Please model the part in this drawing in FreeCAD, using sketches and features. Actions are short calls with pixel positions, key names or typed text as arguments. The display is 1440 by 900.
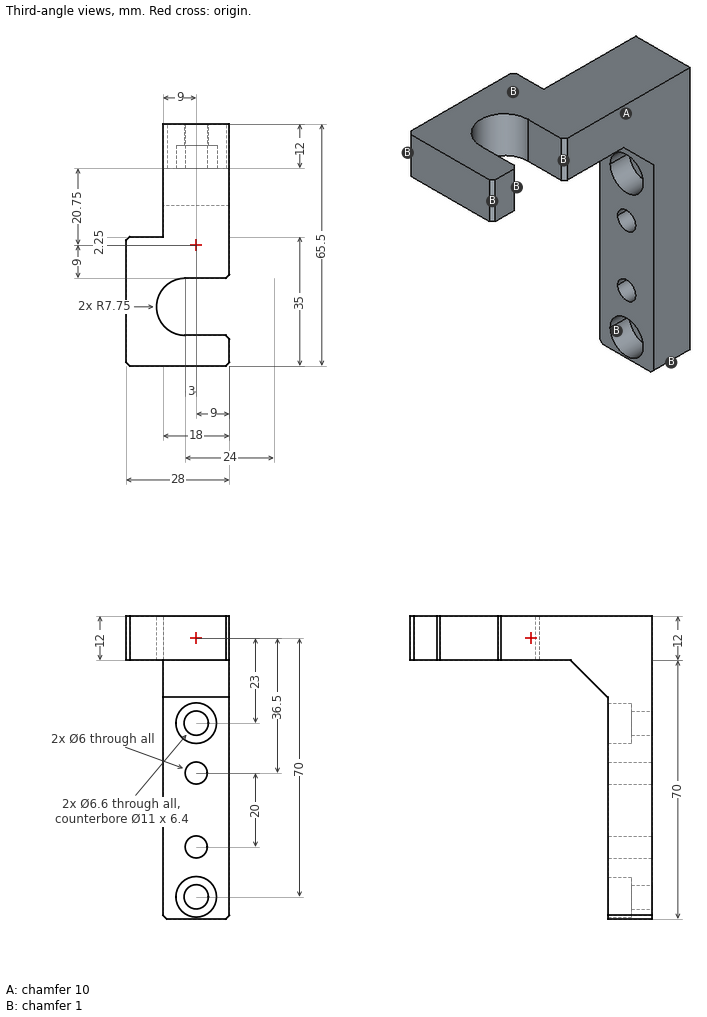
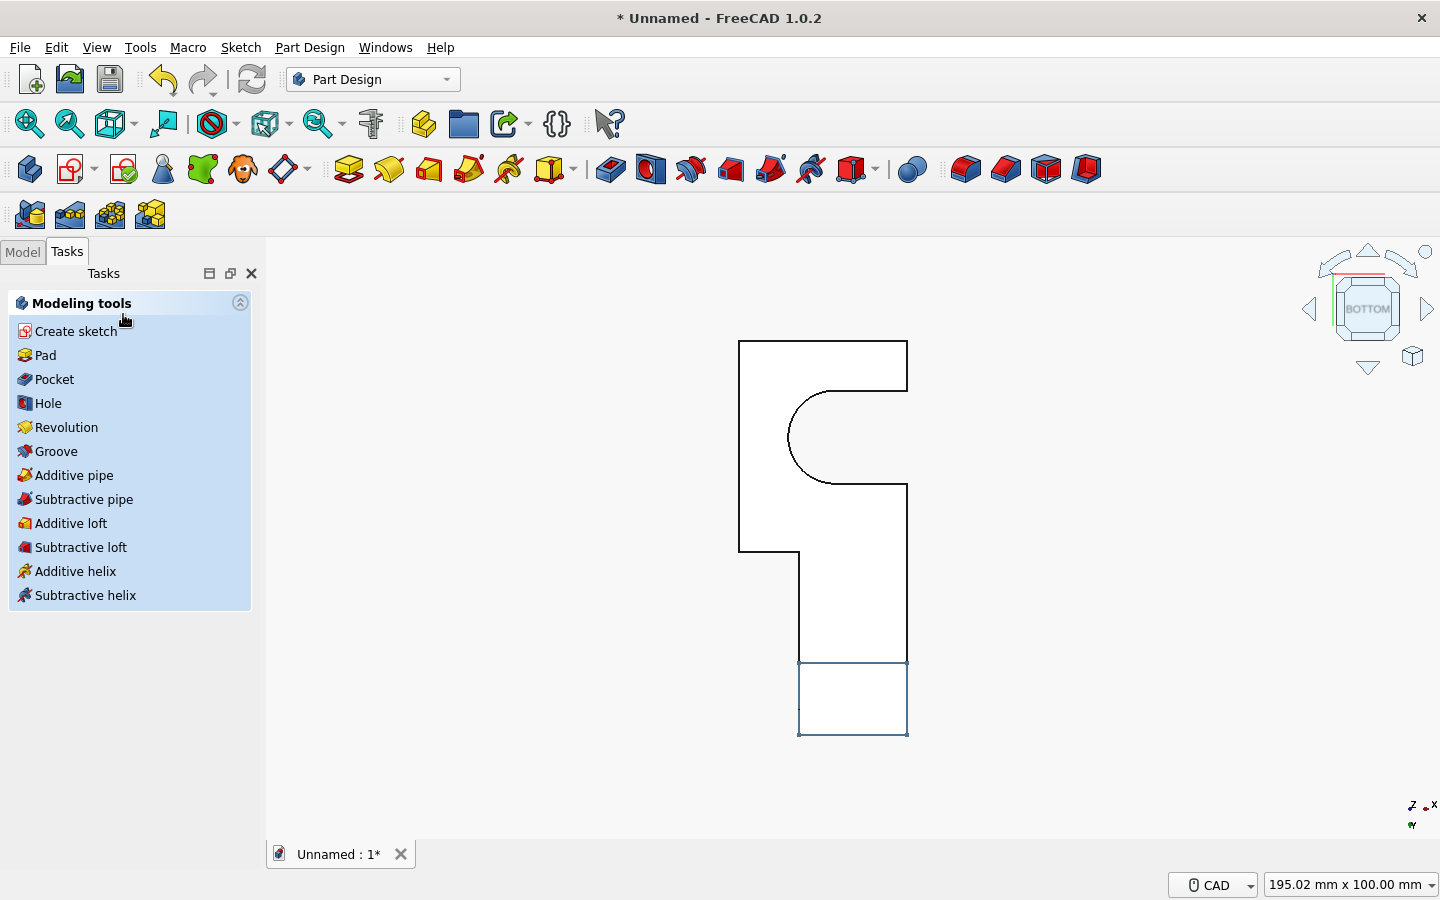
click(350, 170)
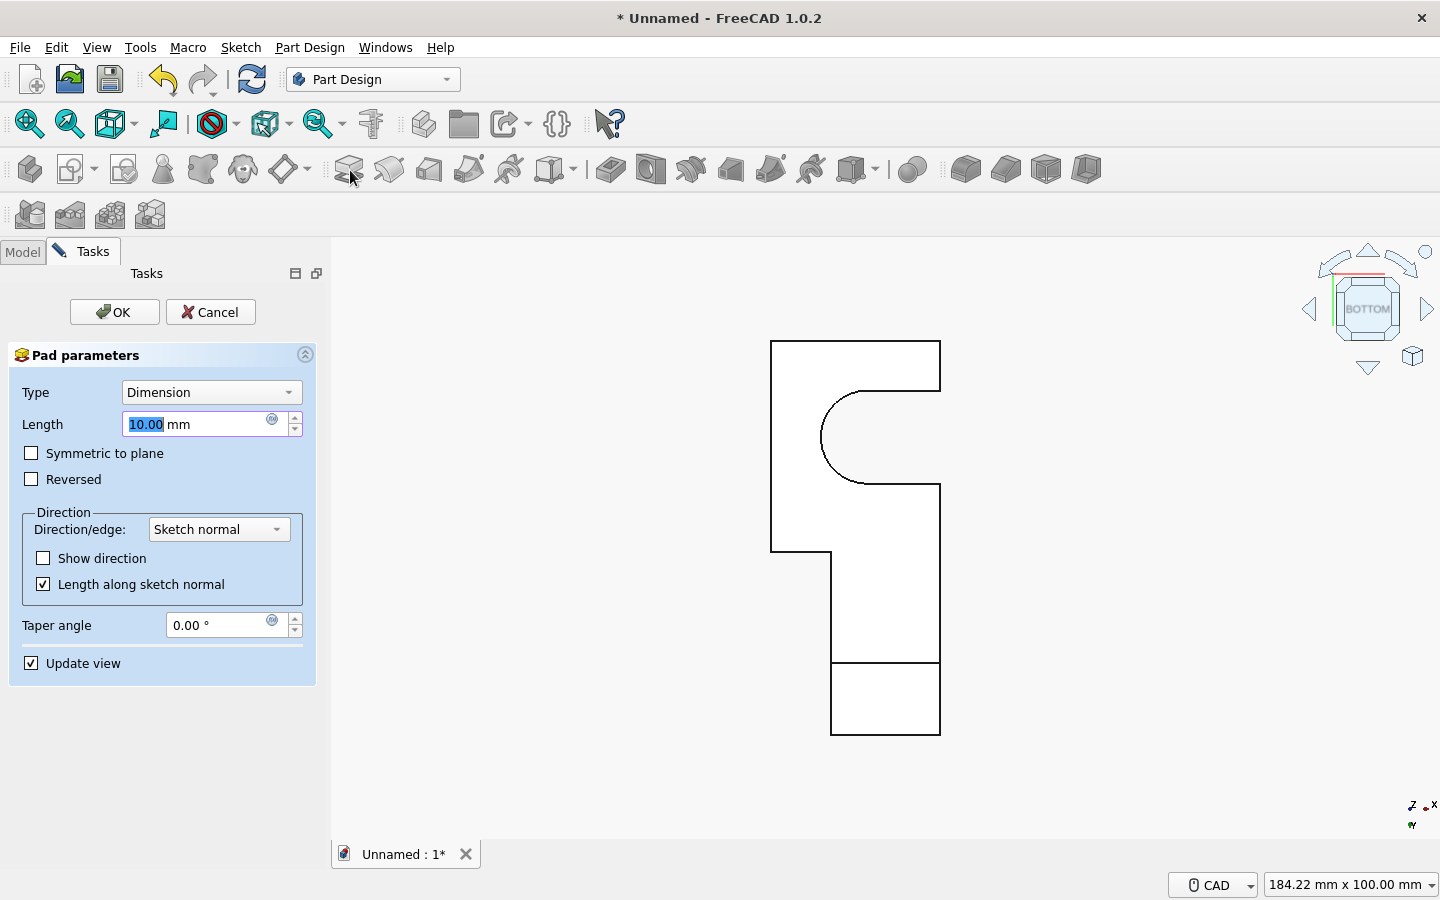
text(70)
key(Tab)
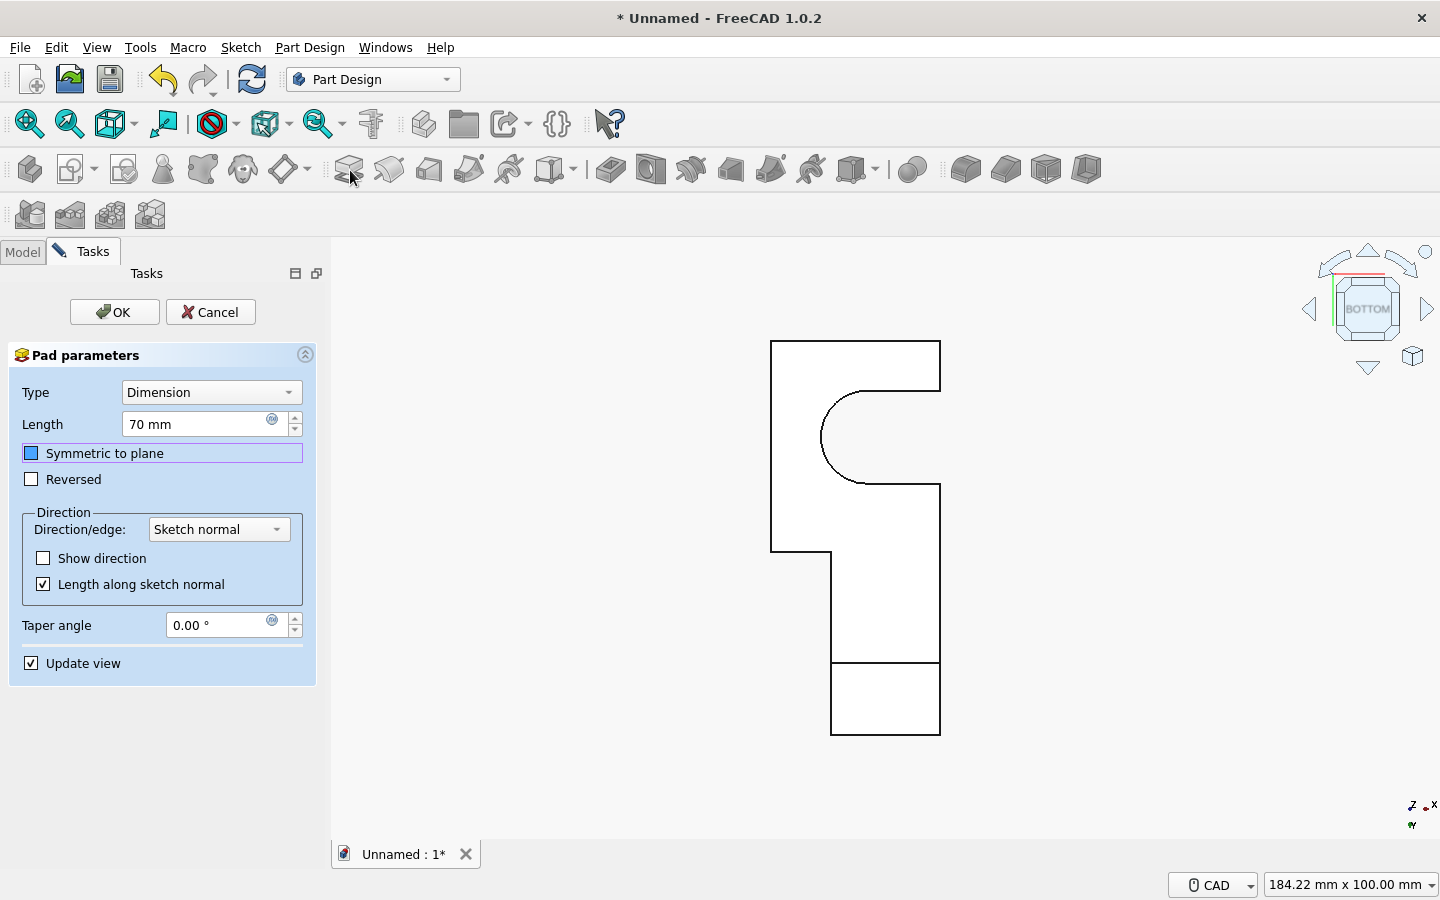
click(115, 312)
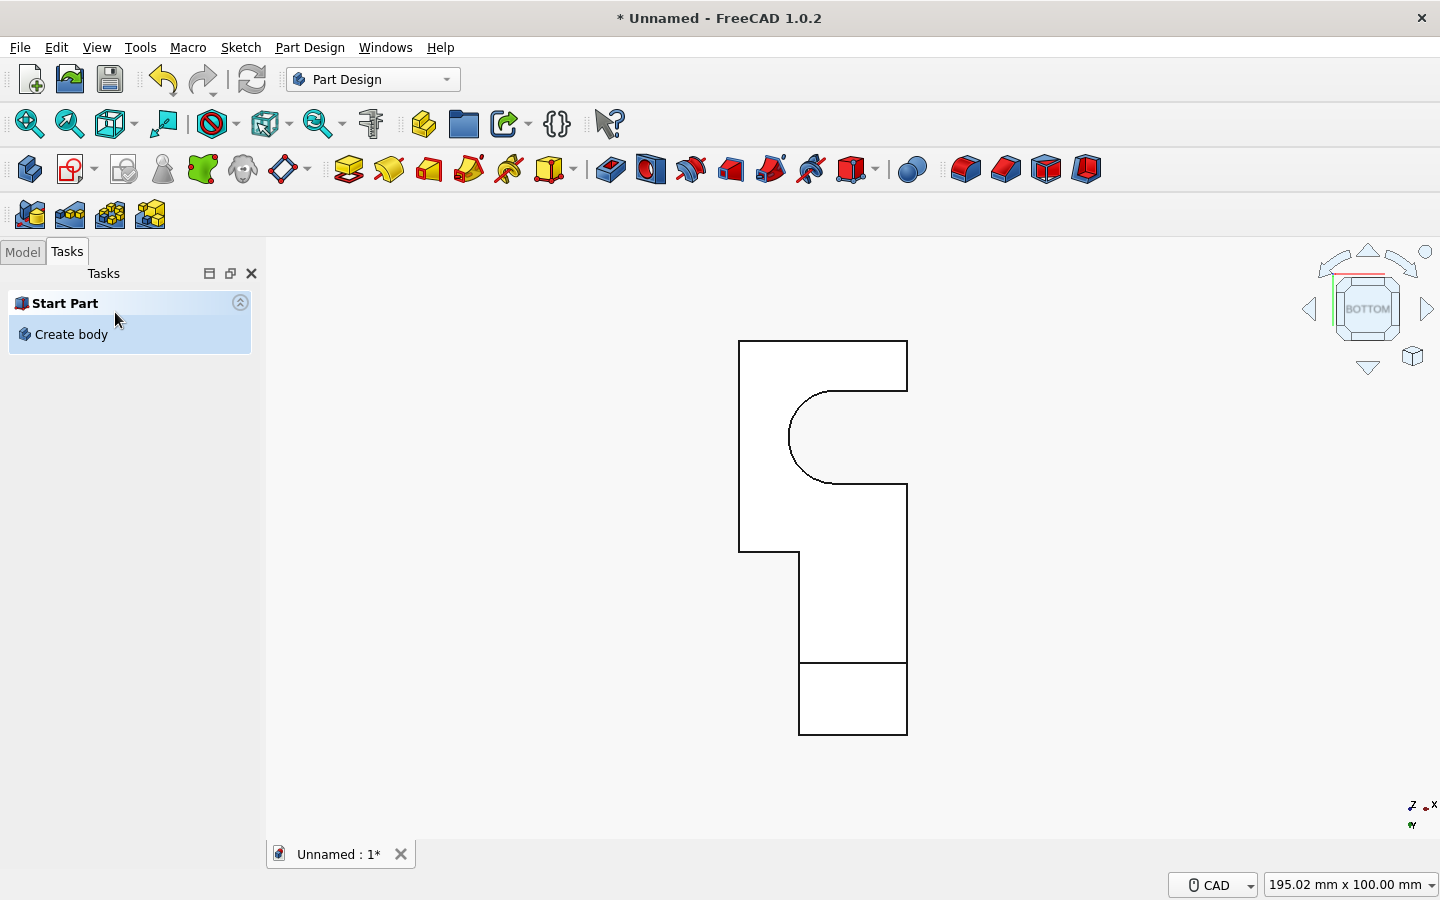
key(0)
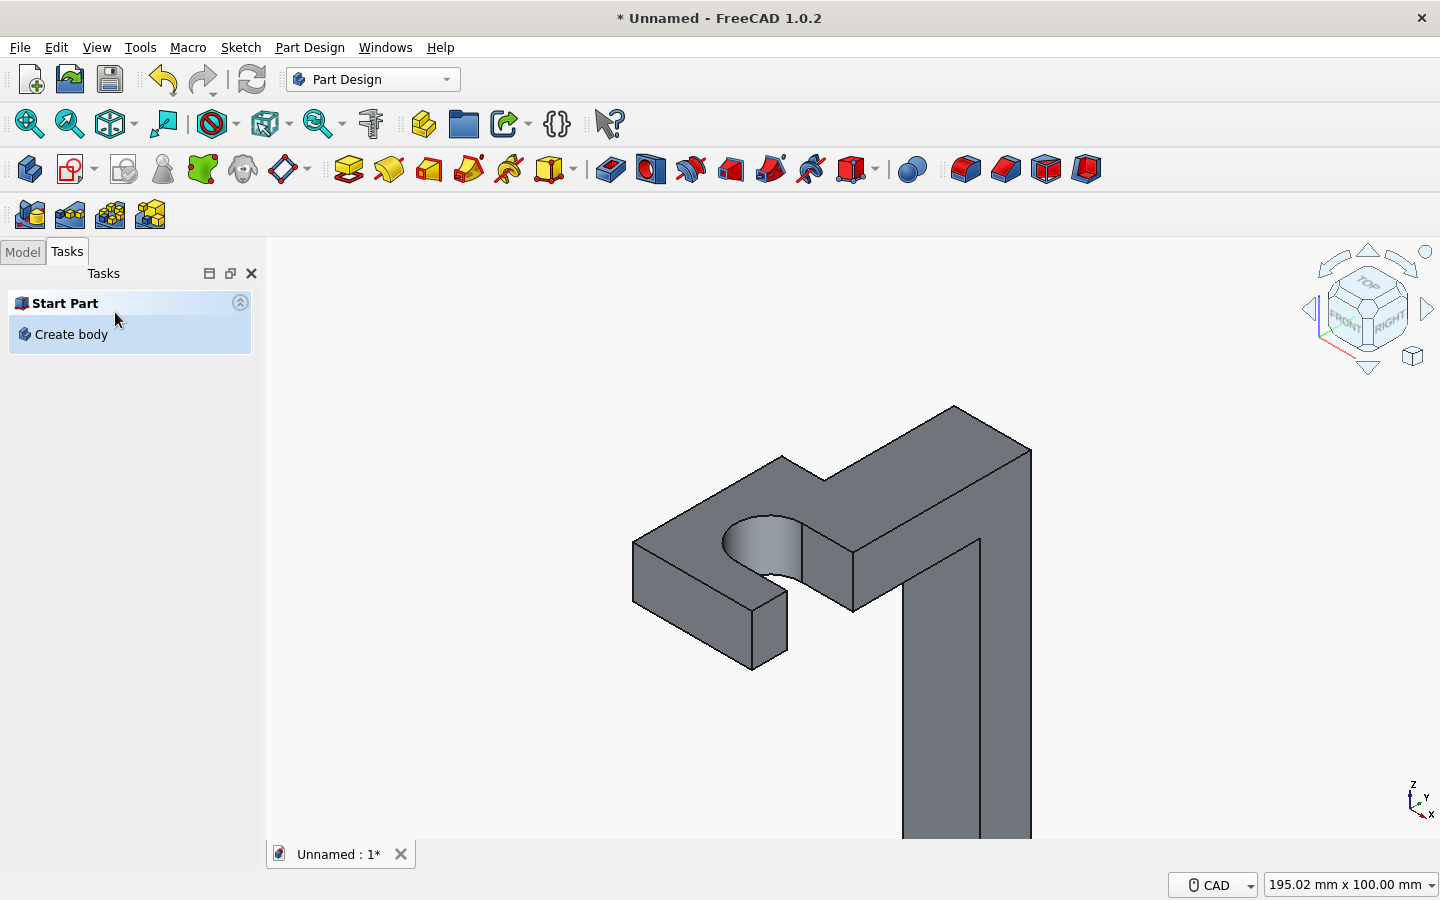
click(30, 124)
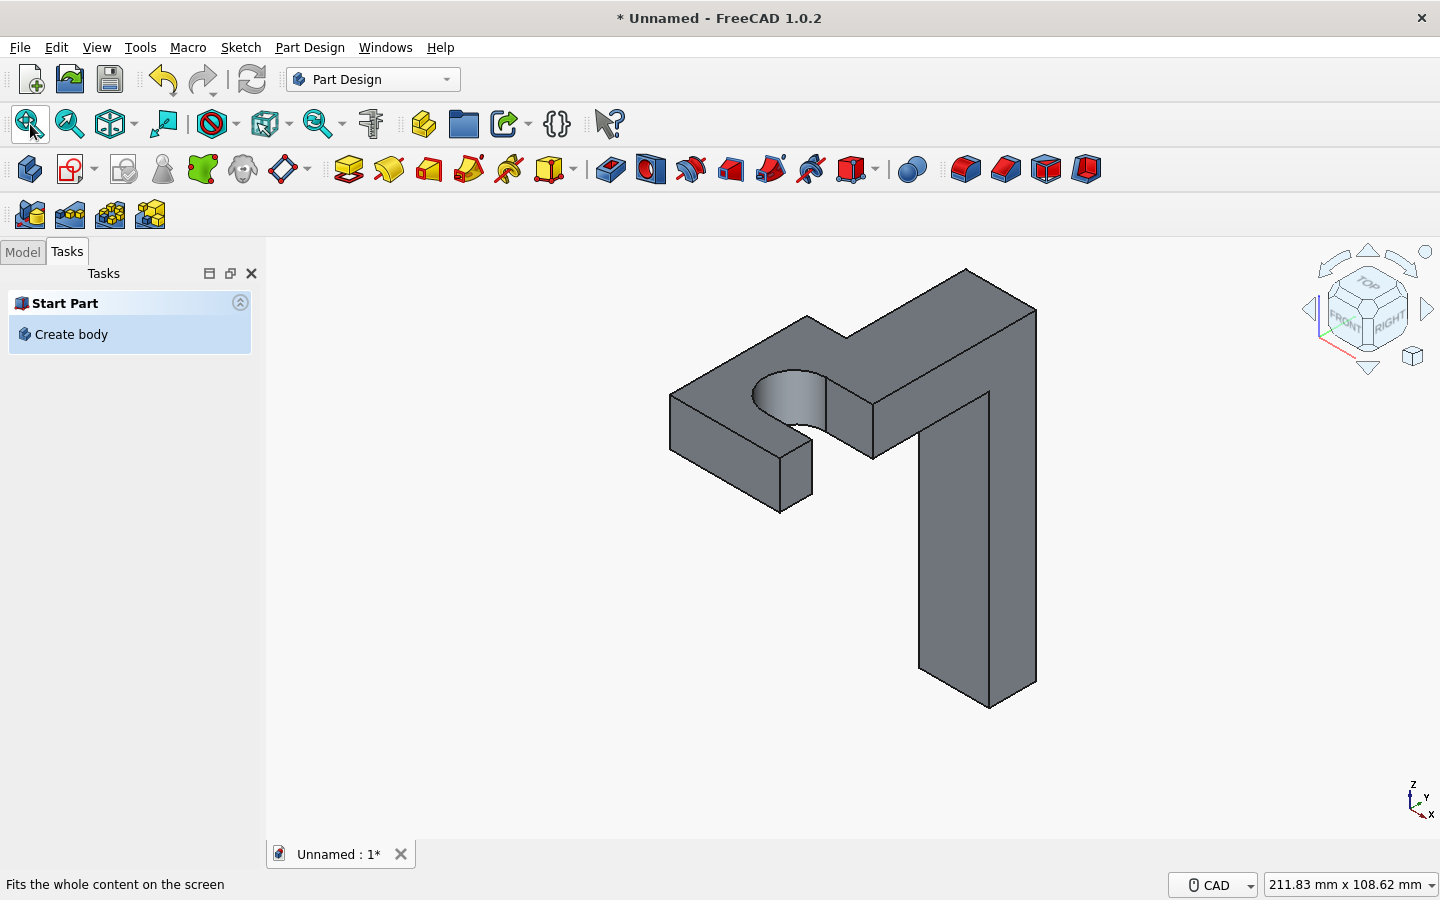
key(2)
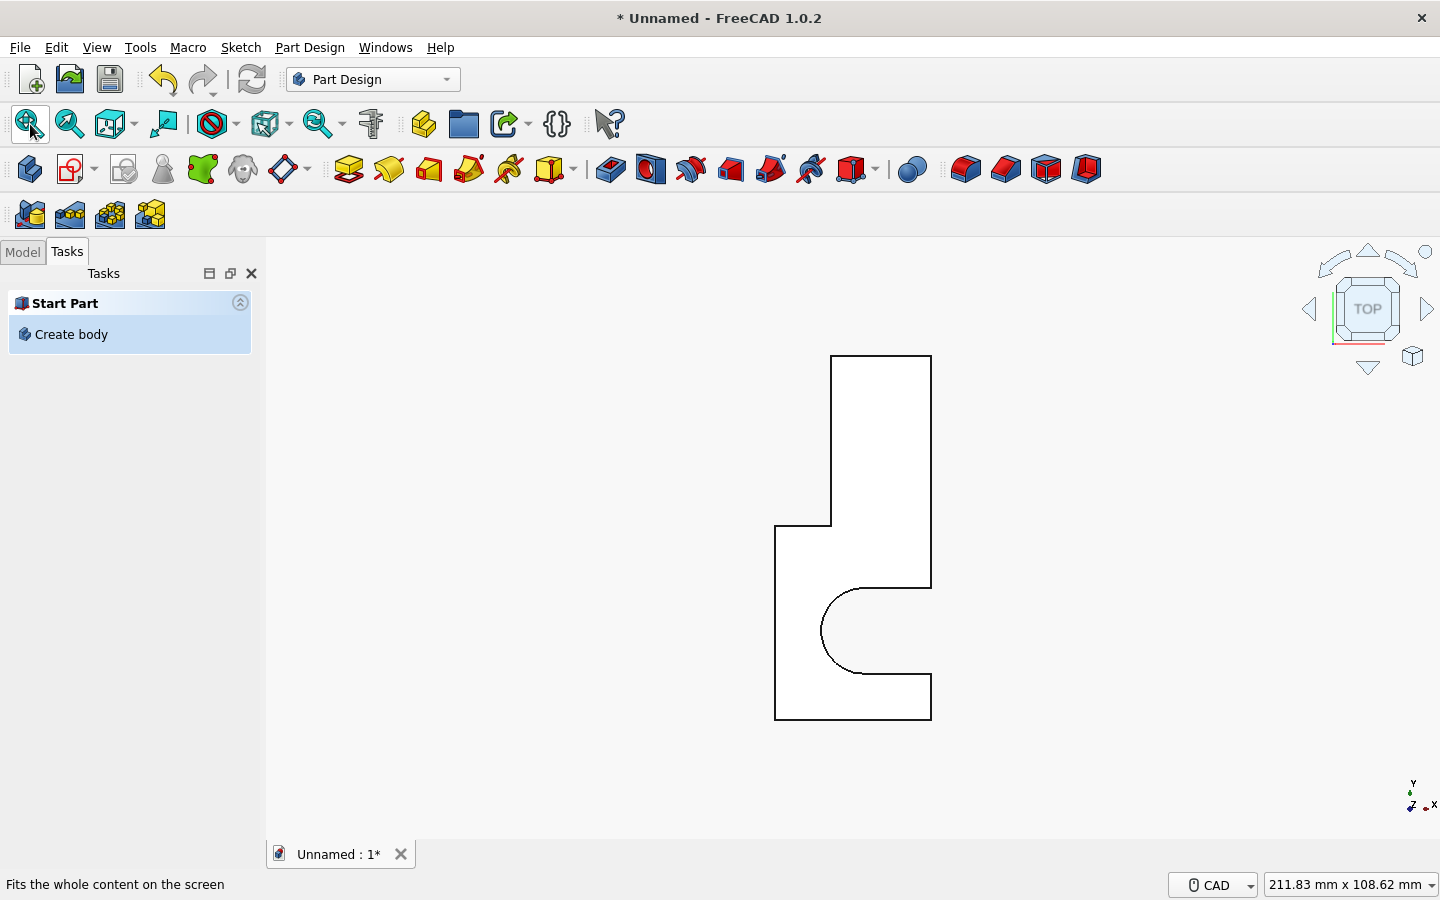
key(1)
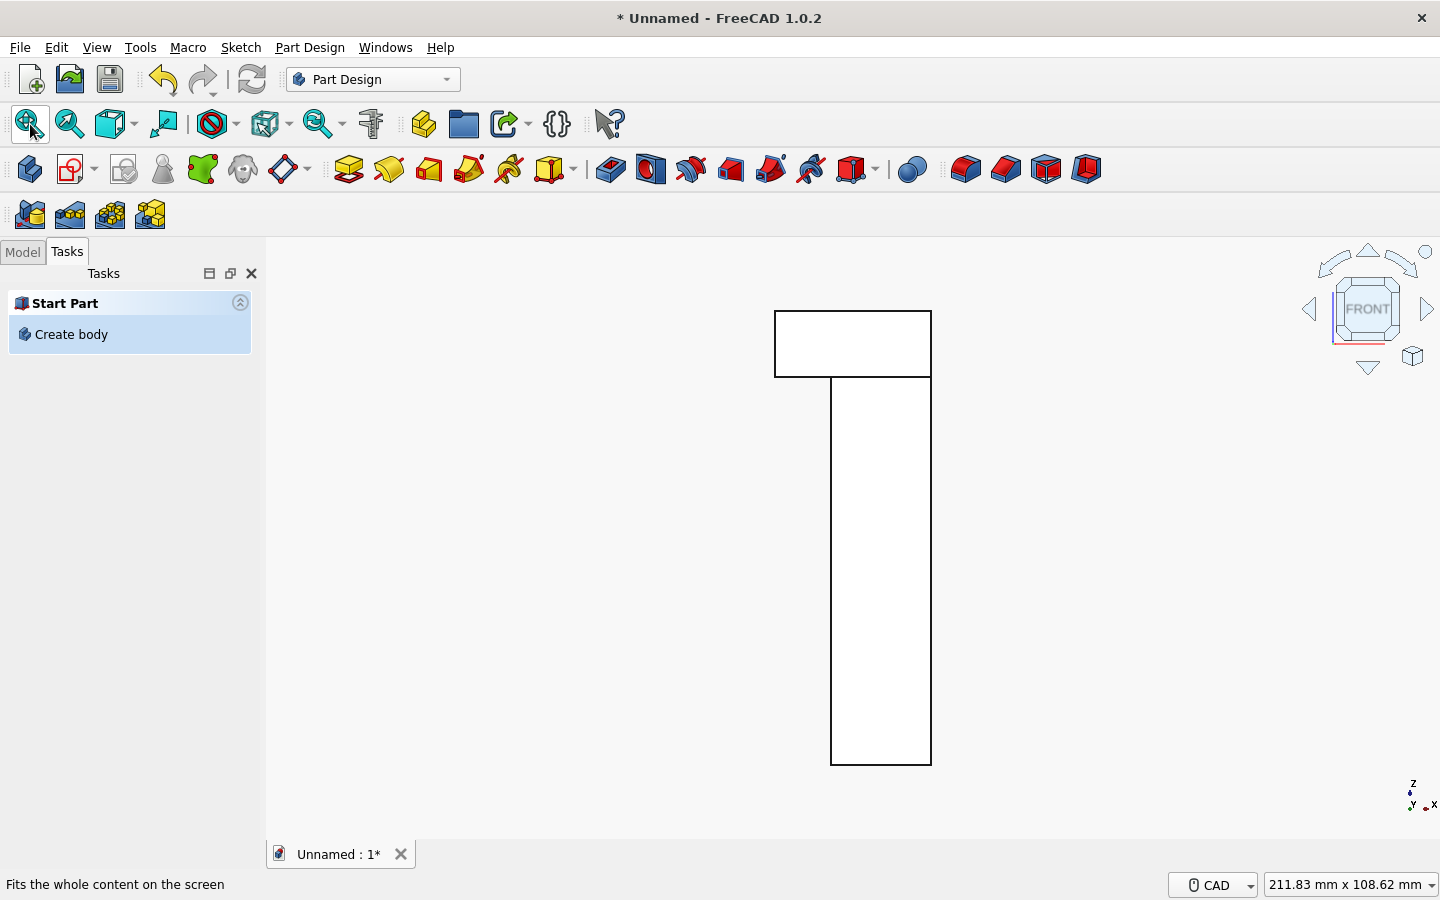
key(3)